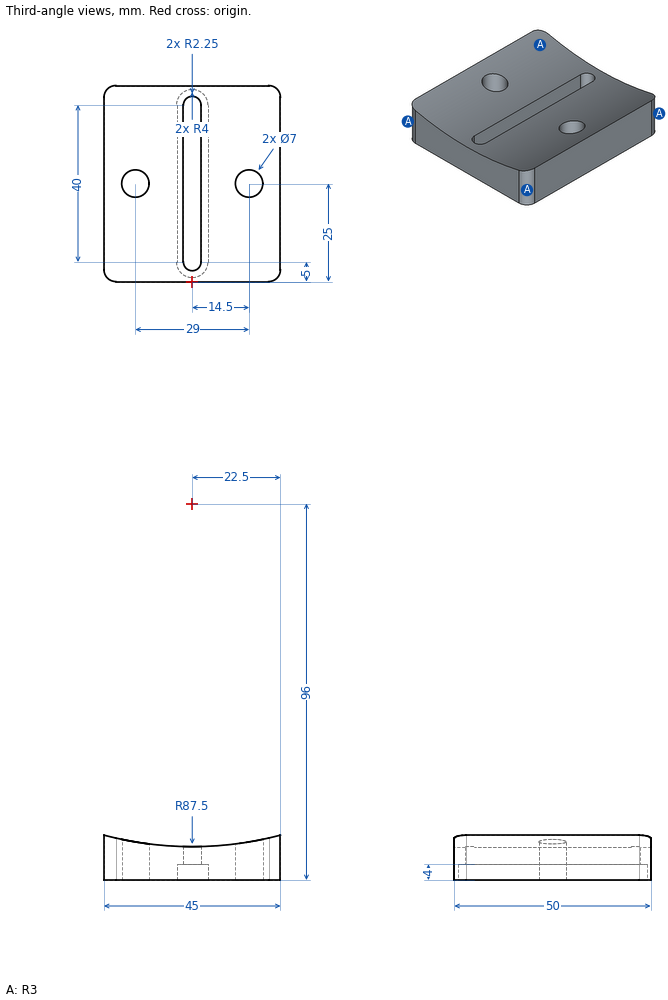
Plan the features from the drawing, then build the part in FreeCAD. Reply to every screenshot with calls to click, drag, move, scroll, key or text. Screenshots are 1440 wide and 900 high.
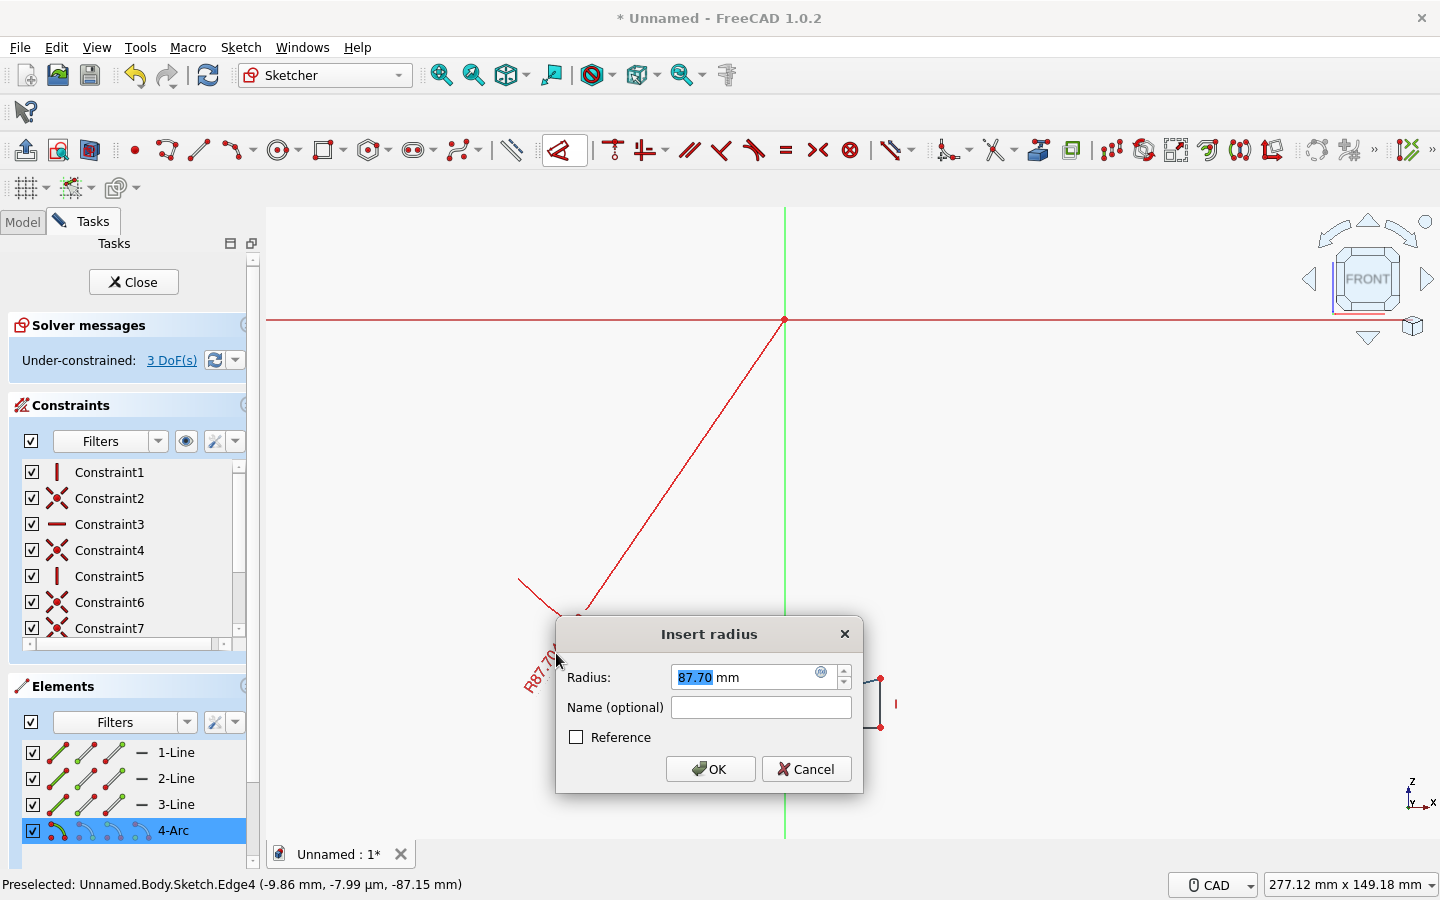
text(87.5)
key(Return)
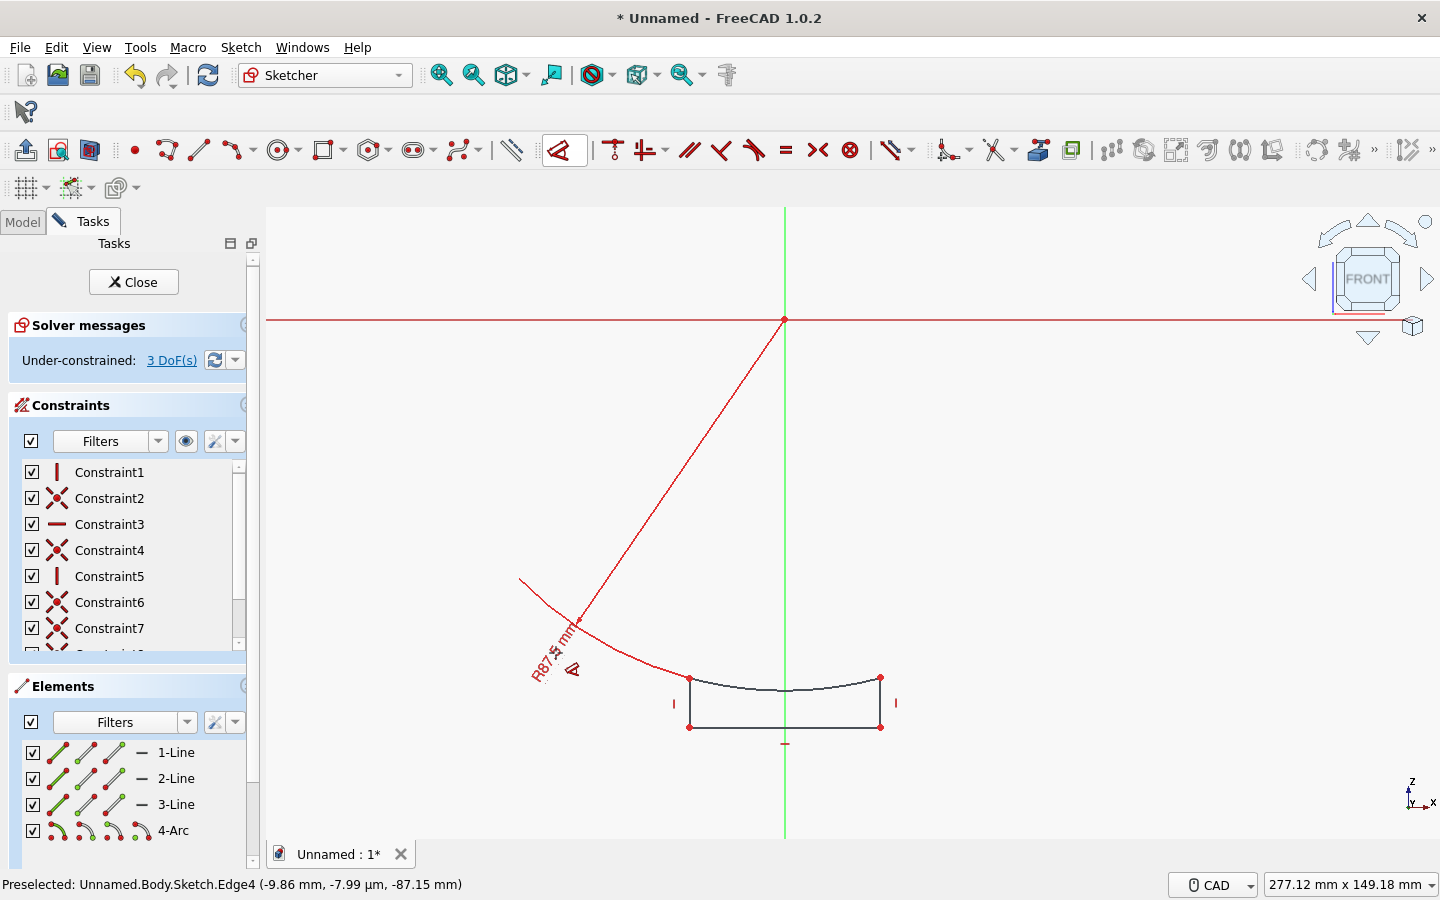
click(823, 728)
click(741, 762)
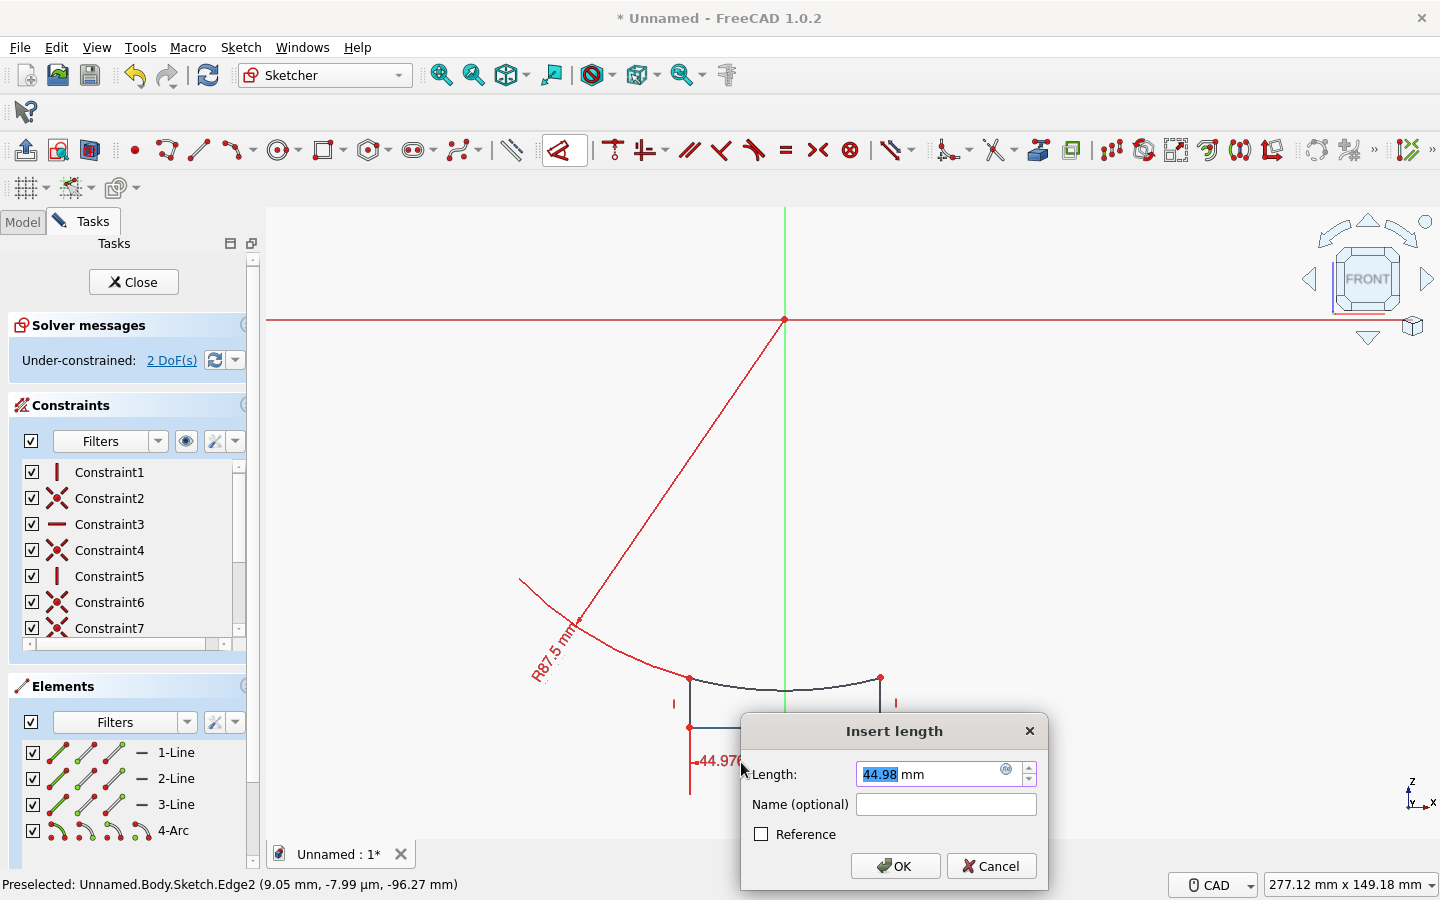
text(45)
key(Return)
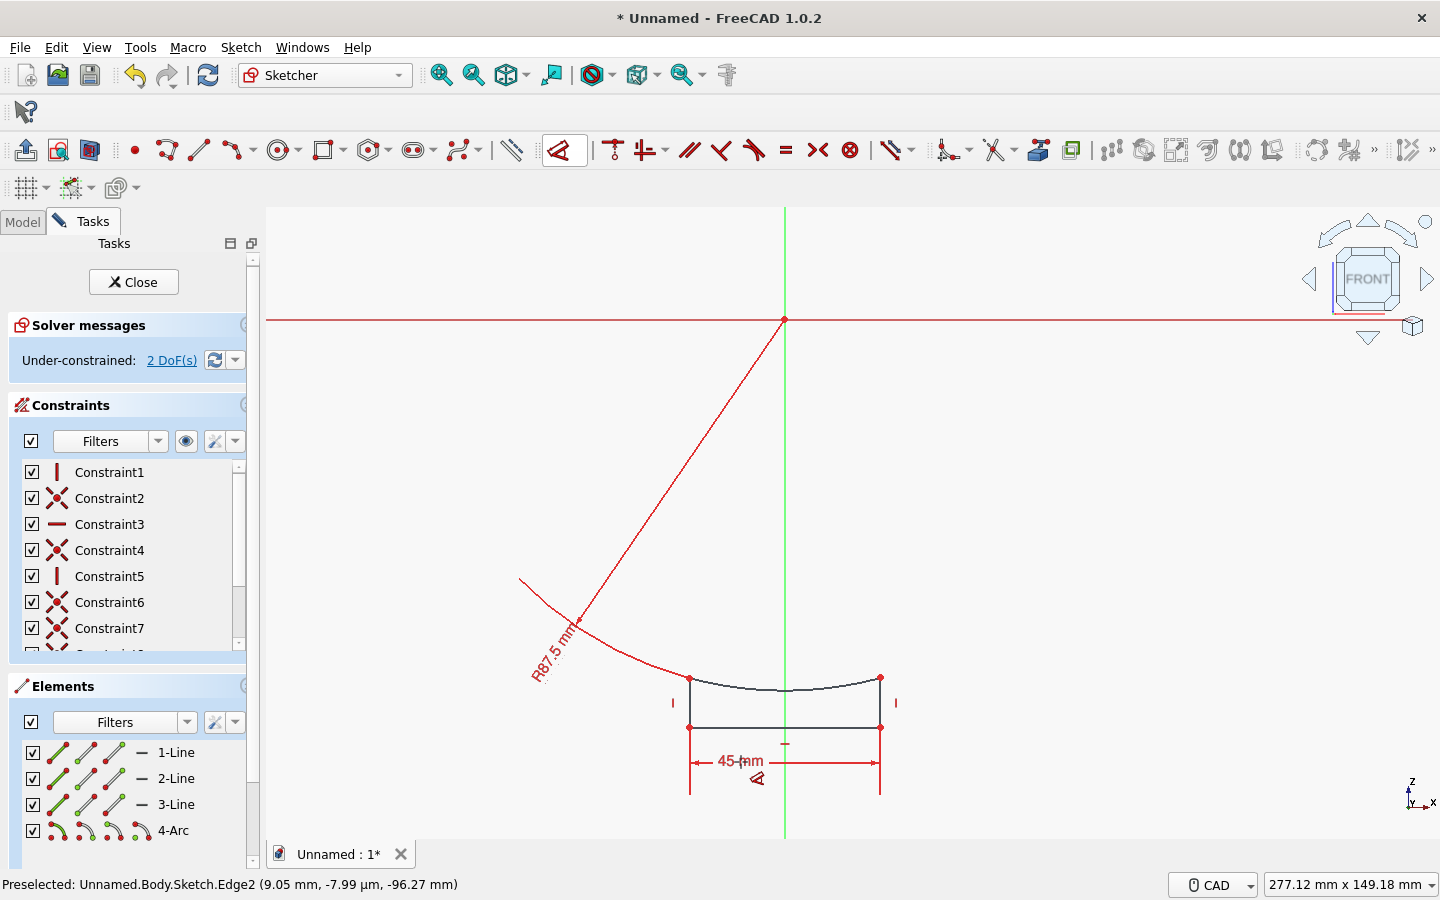
click(880, 728)
click(914, 524)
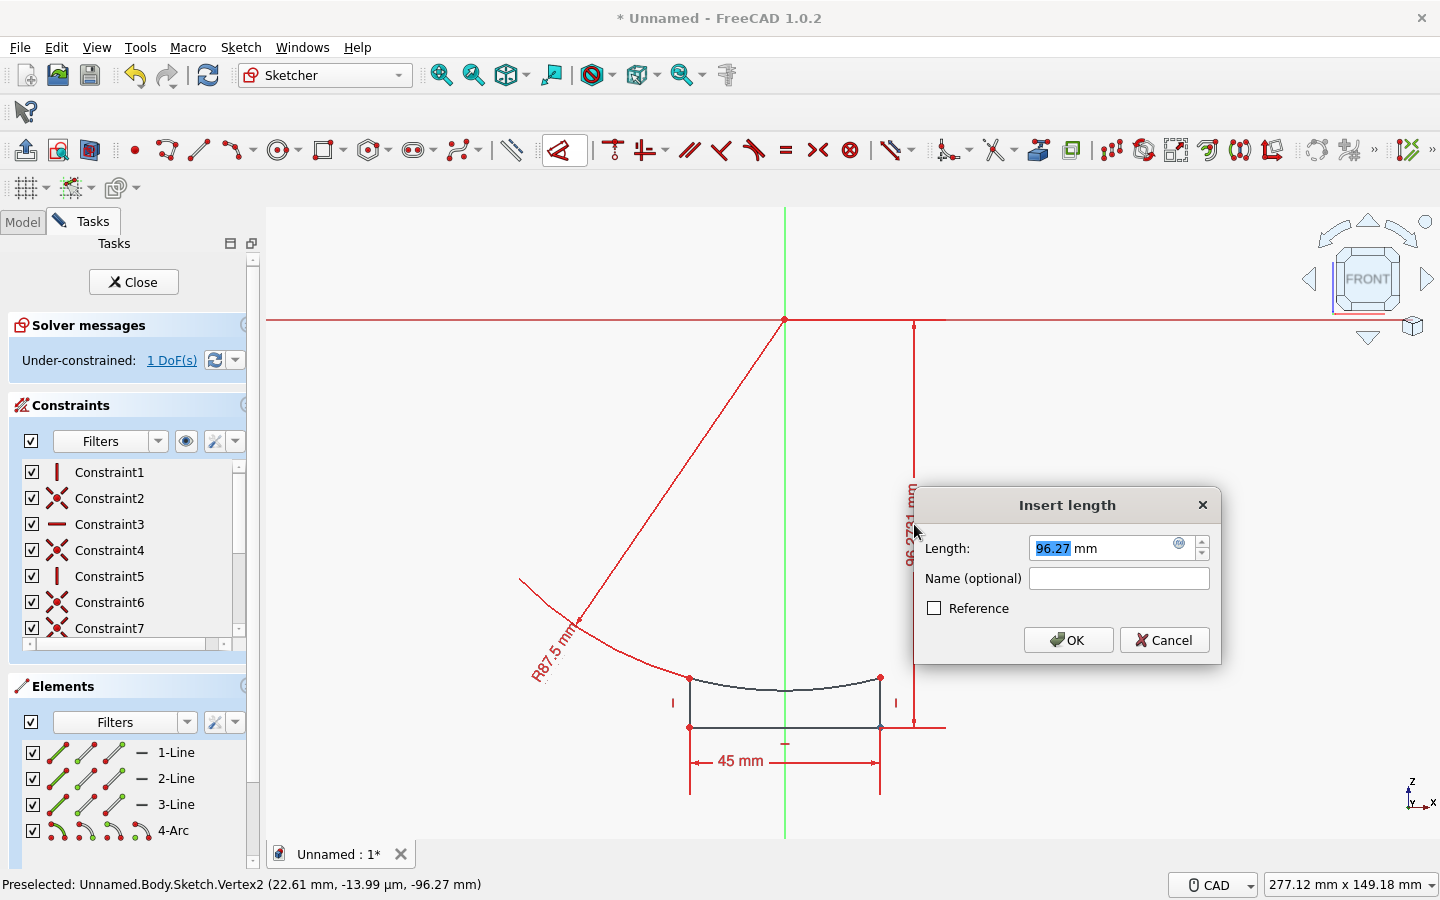
text(96)
key(Return)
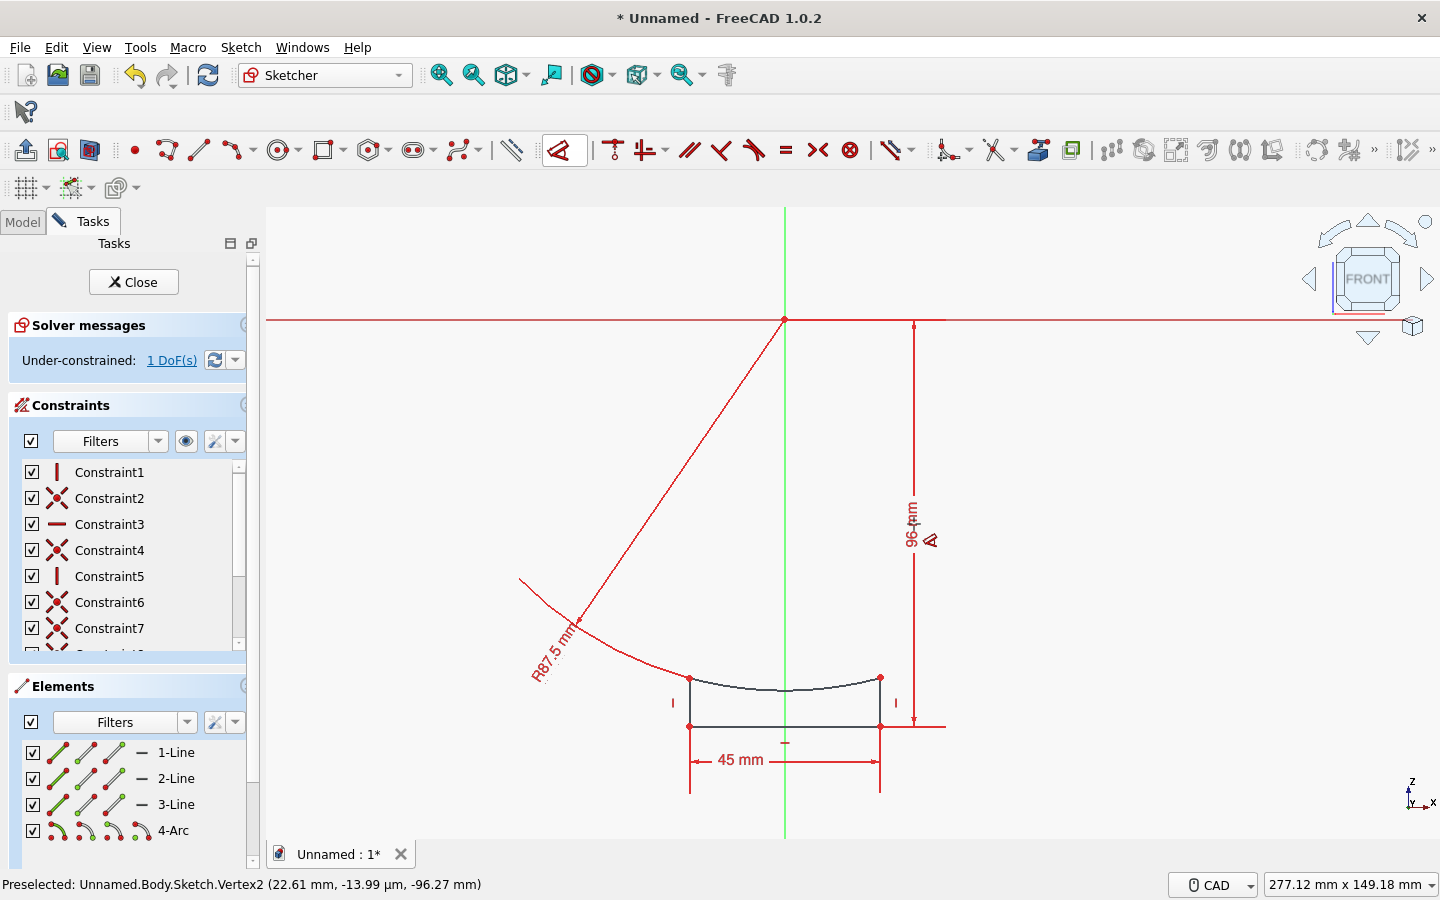
click(880, 678)
click(833, 286)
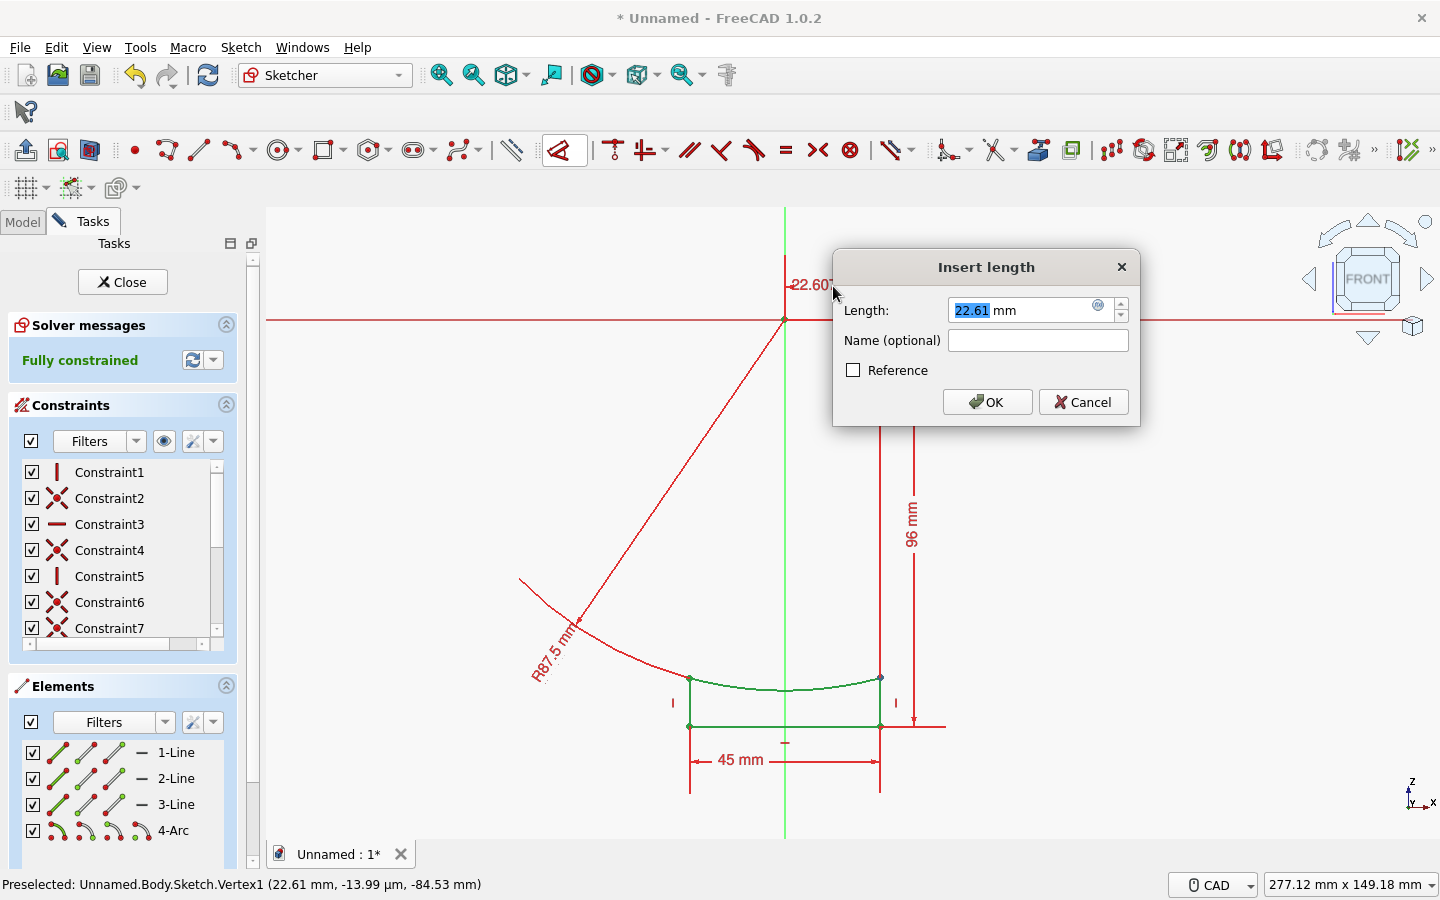
text(22.5)
key(Return)
key(Escape)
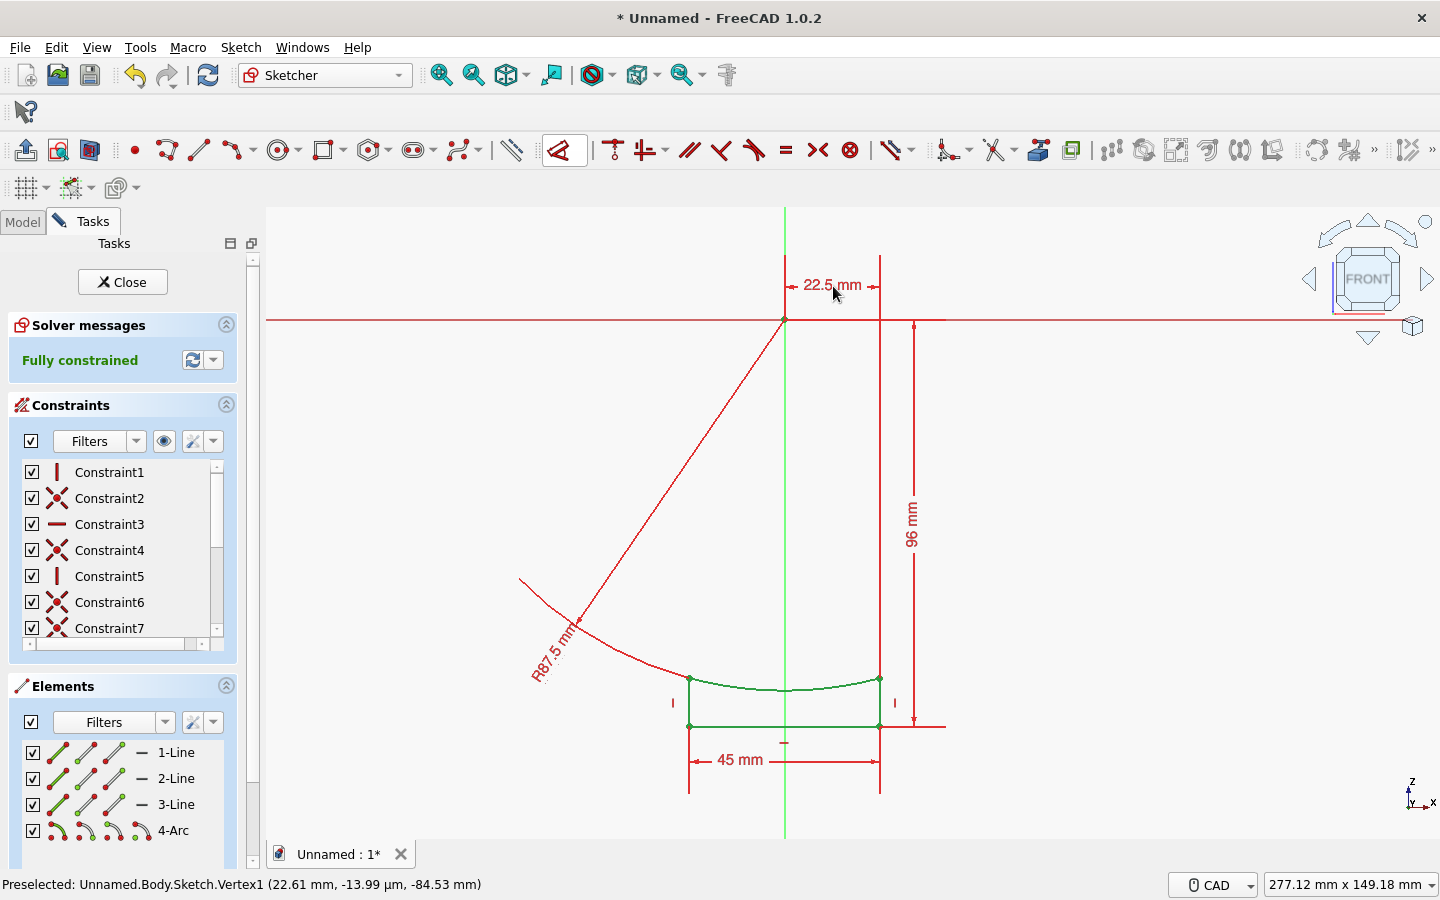
click(123, 282)